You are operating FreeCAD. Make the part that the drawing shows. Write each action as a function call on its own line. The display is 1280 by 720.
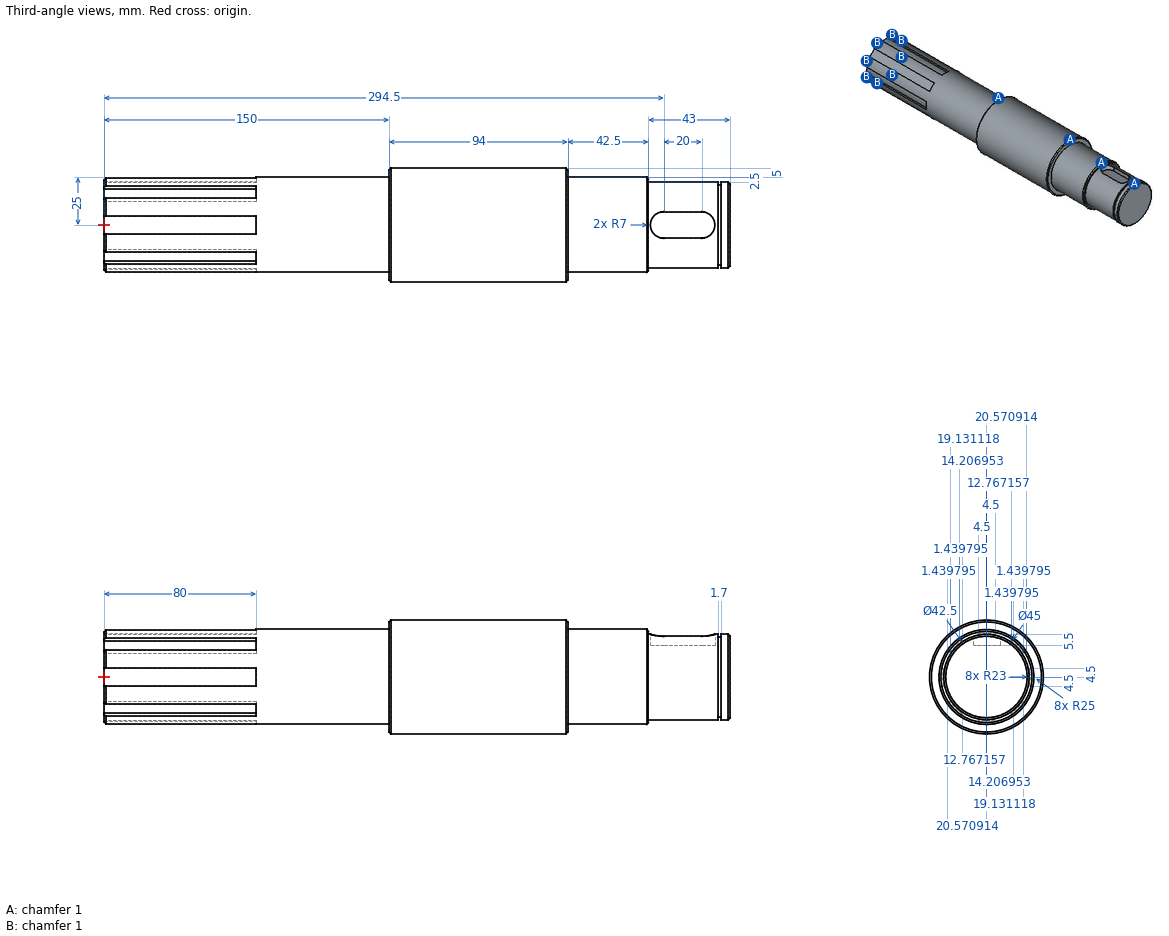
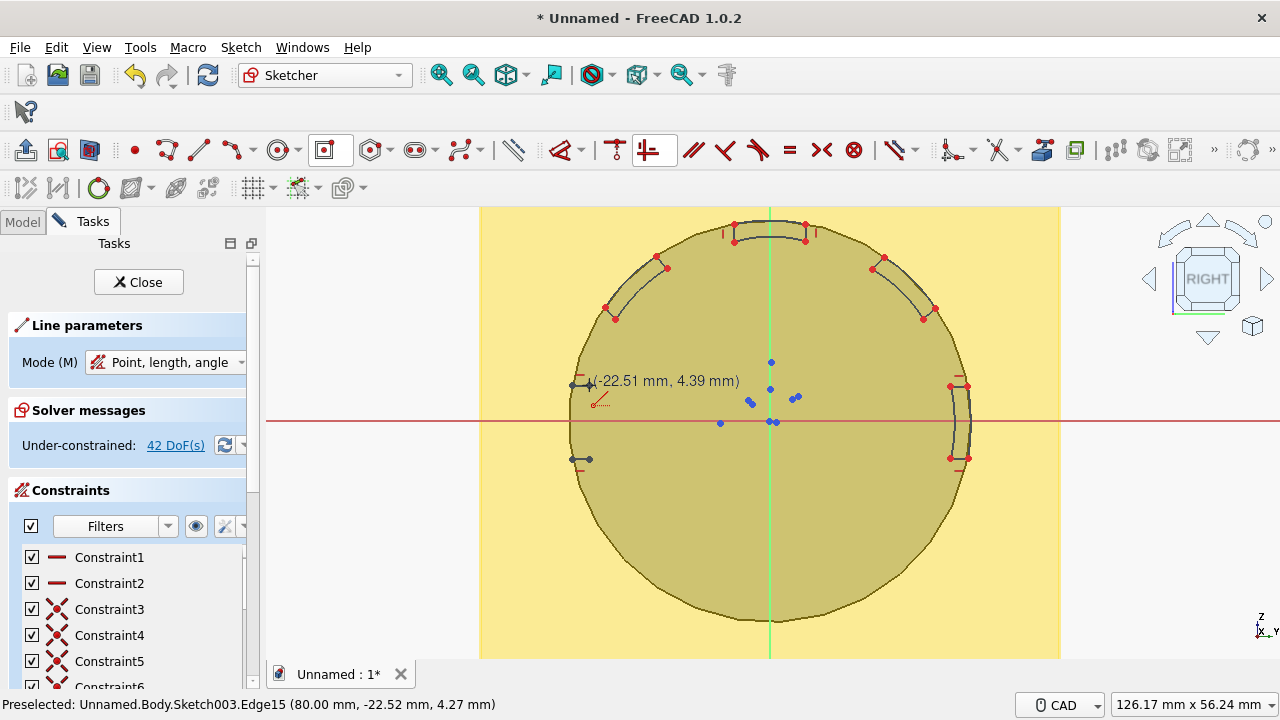
click(232, 150)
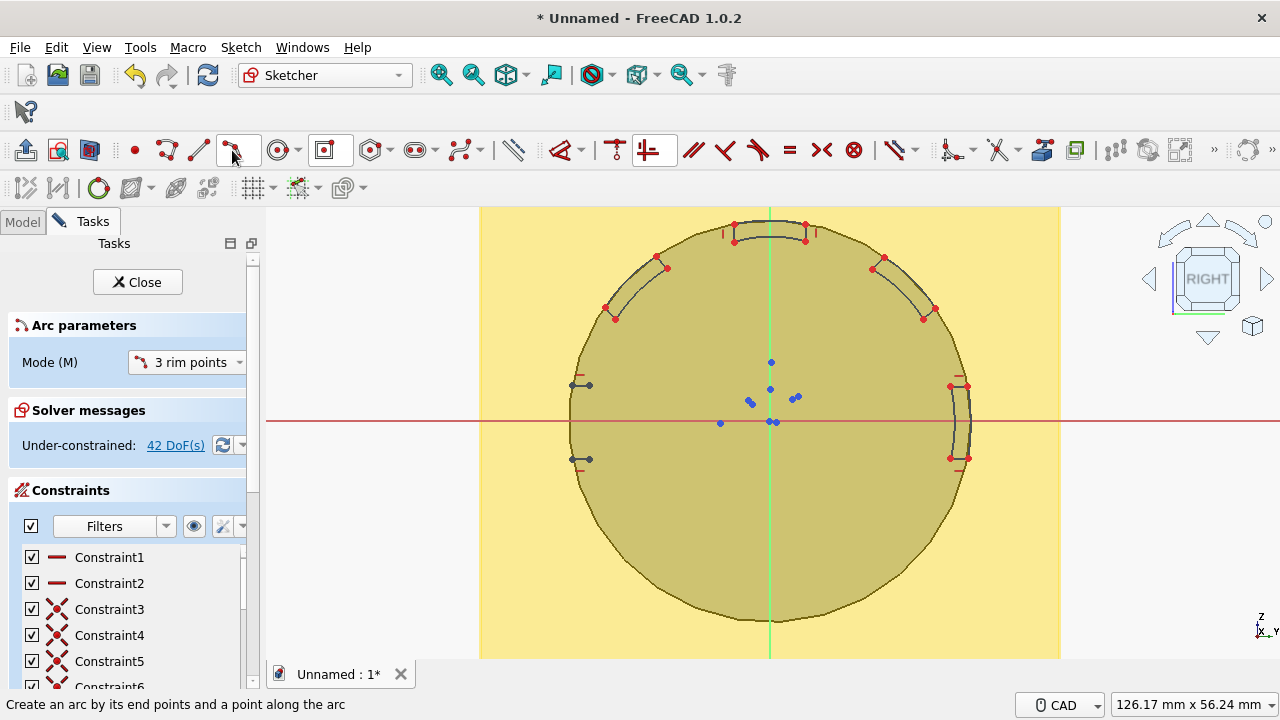
scroll(572, 457, up, 4)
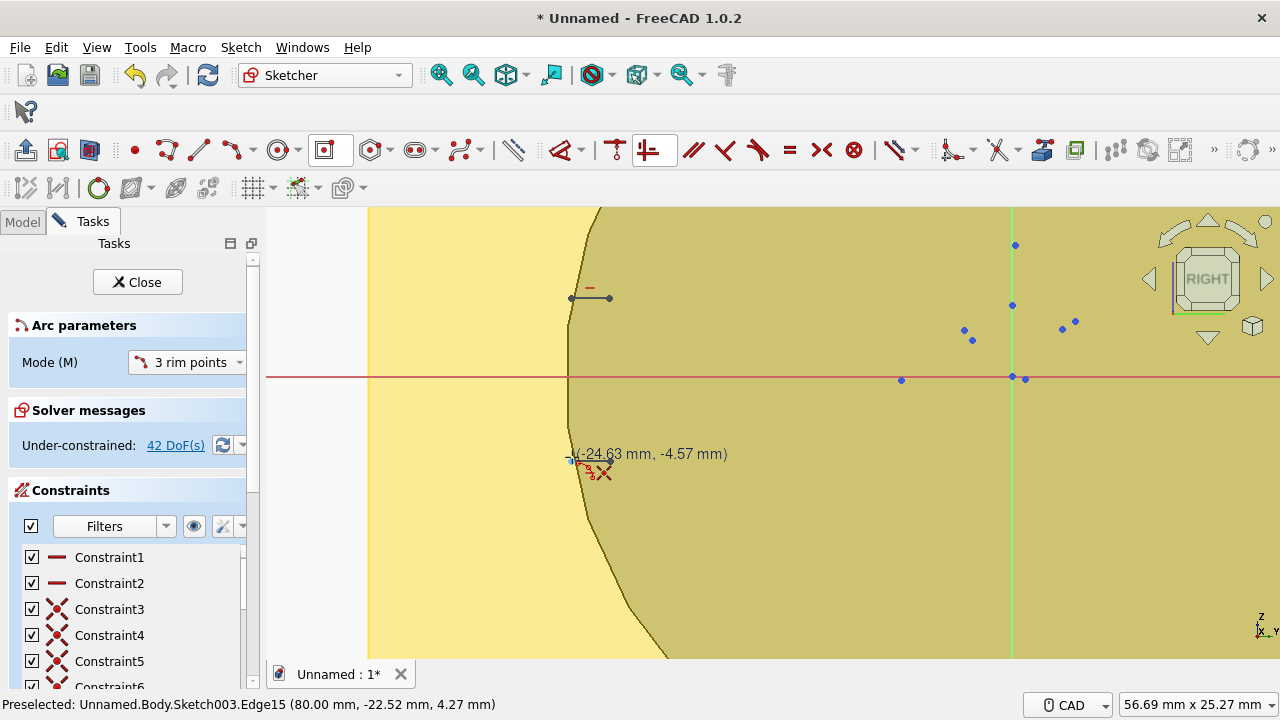
click(572, 461)
click(572, 298)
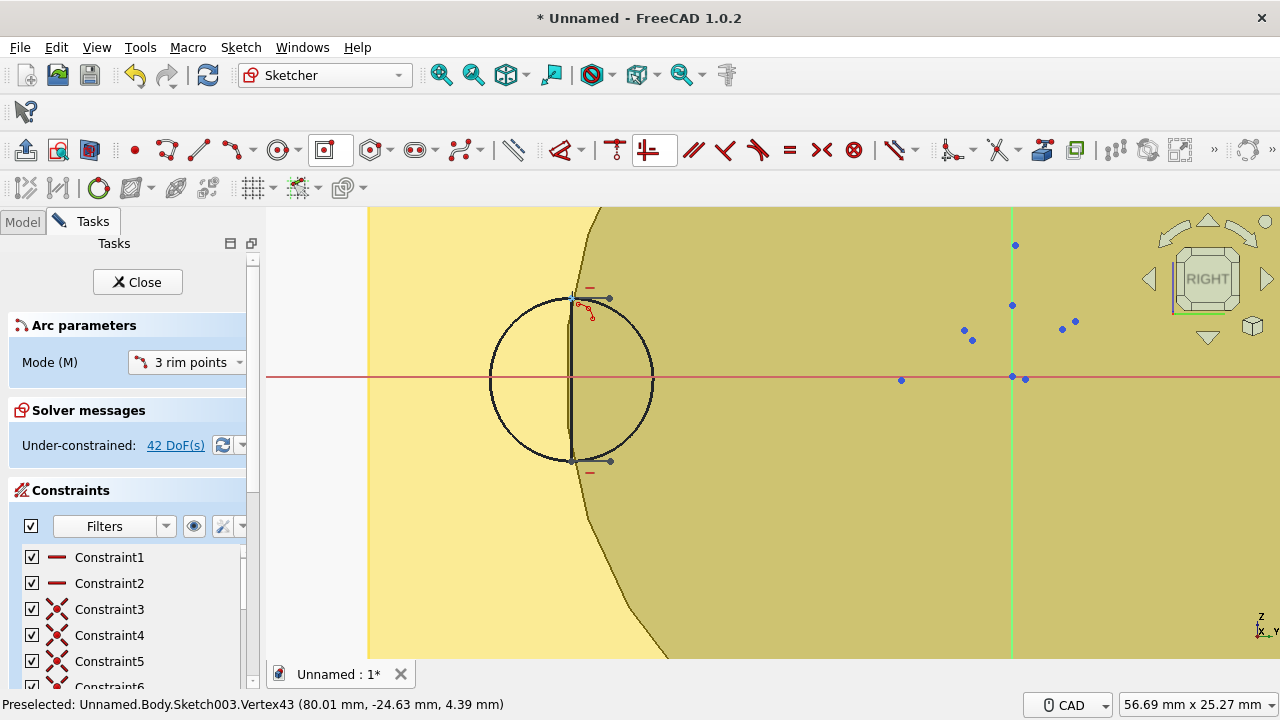
scroll(565, 361, up, 5)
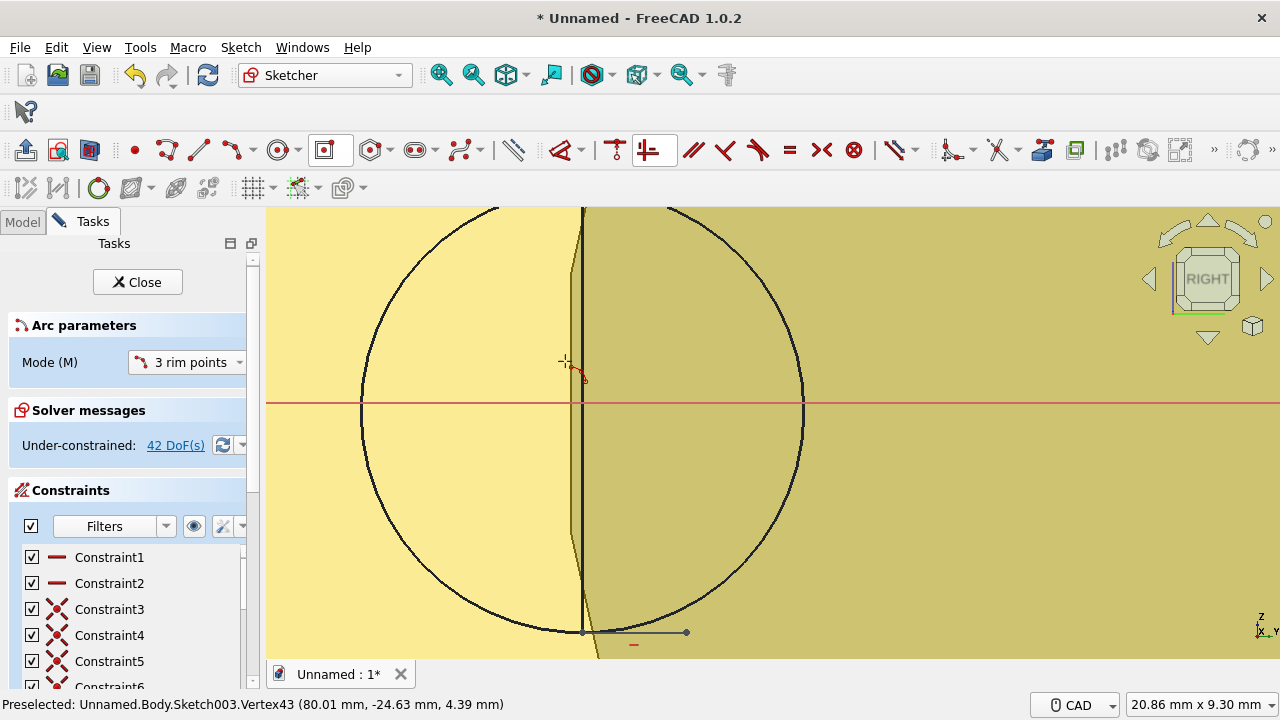
click(565, 359)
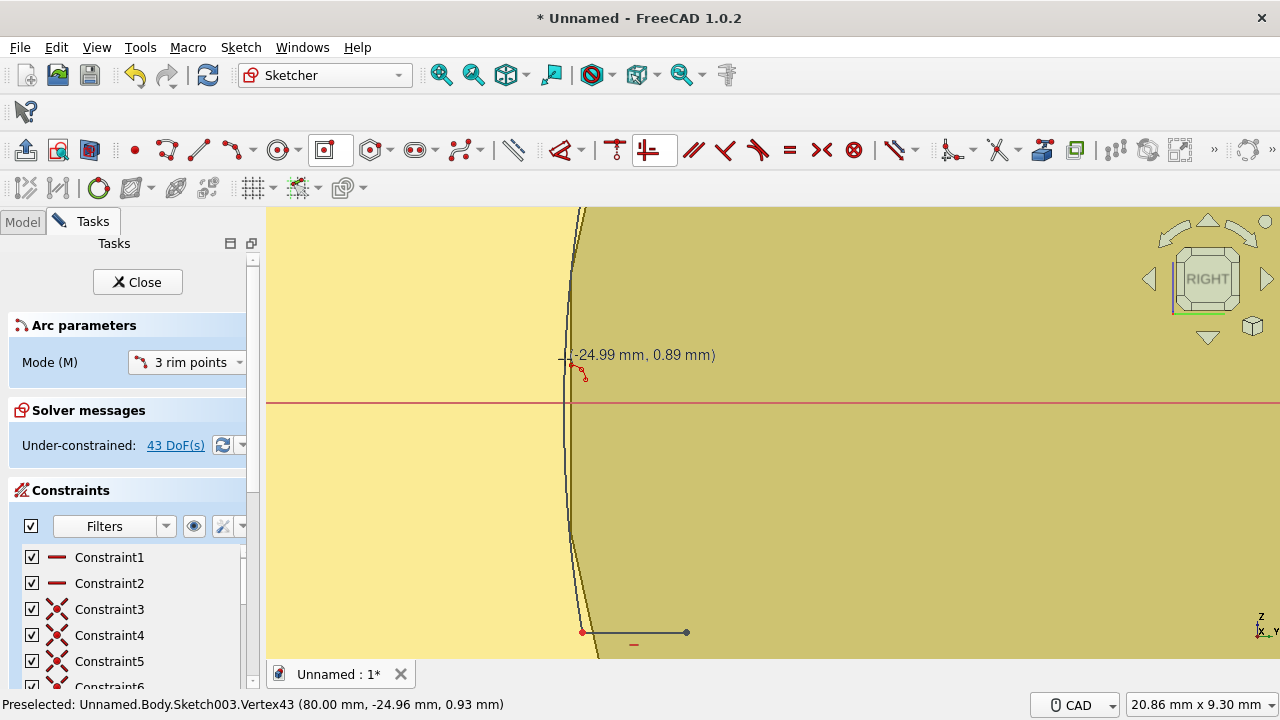
scroll(571, 437, down, 11)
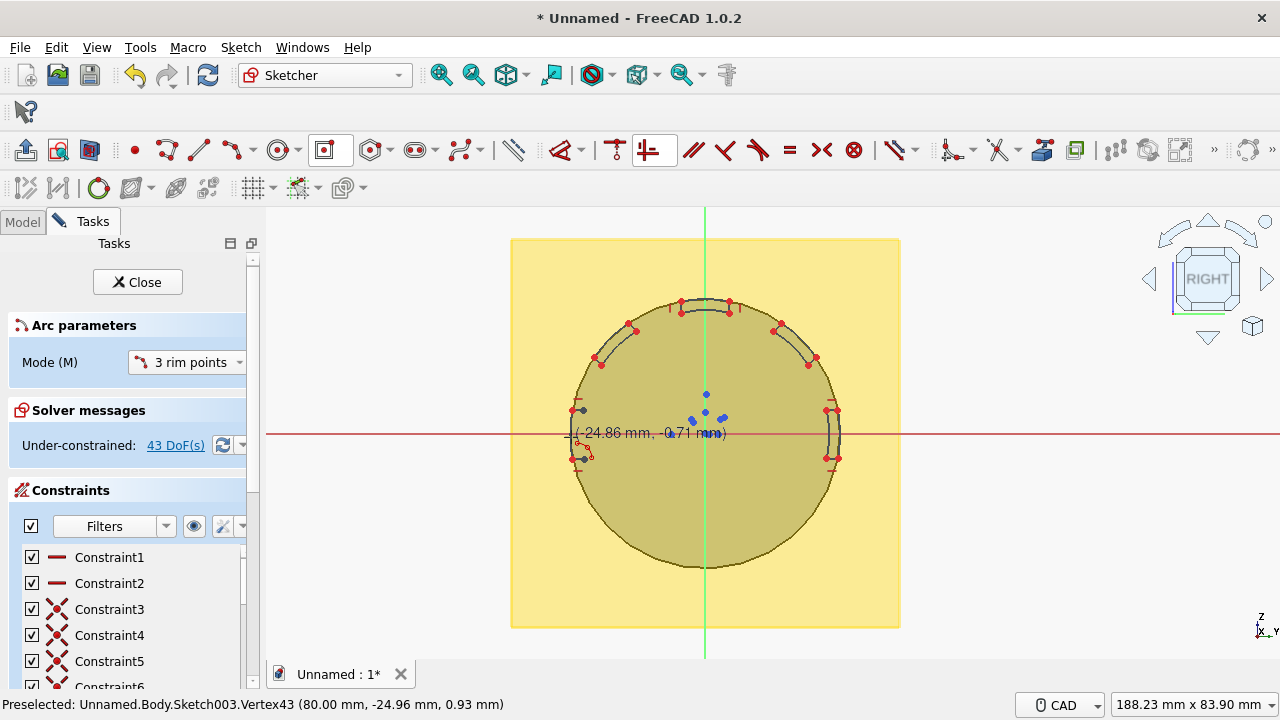
scroll(584, 409, up, 6)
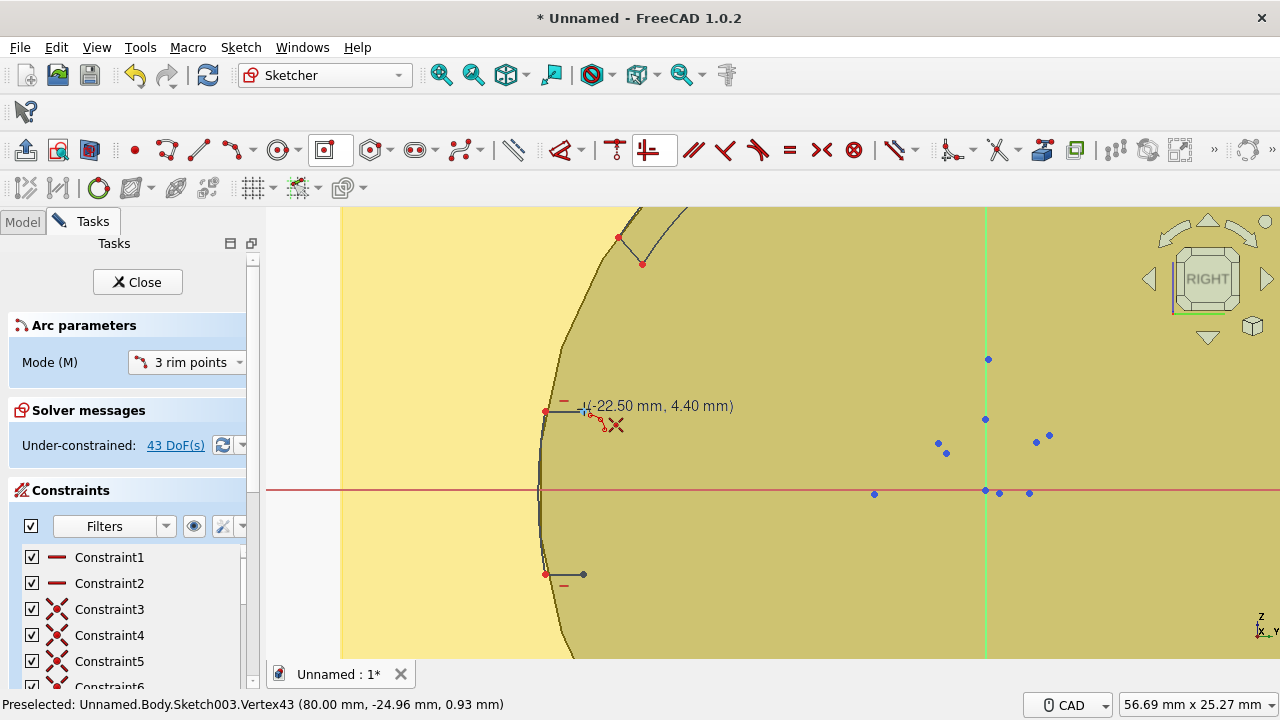
click(583, 412)
click(584, 575)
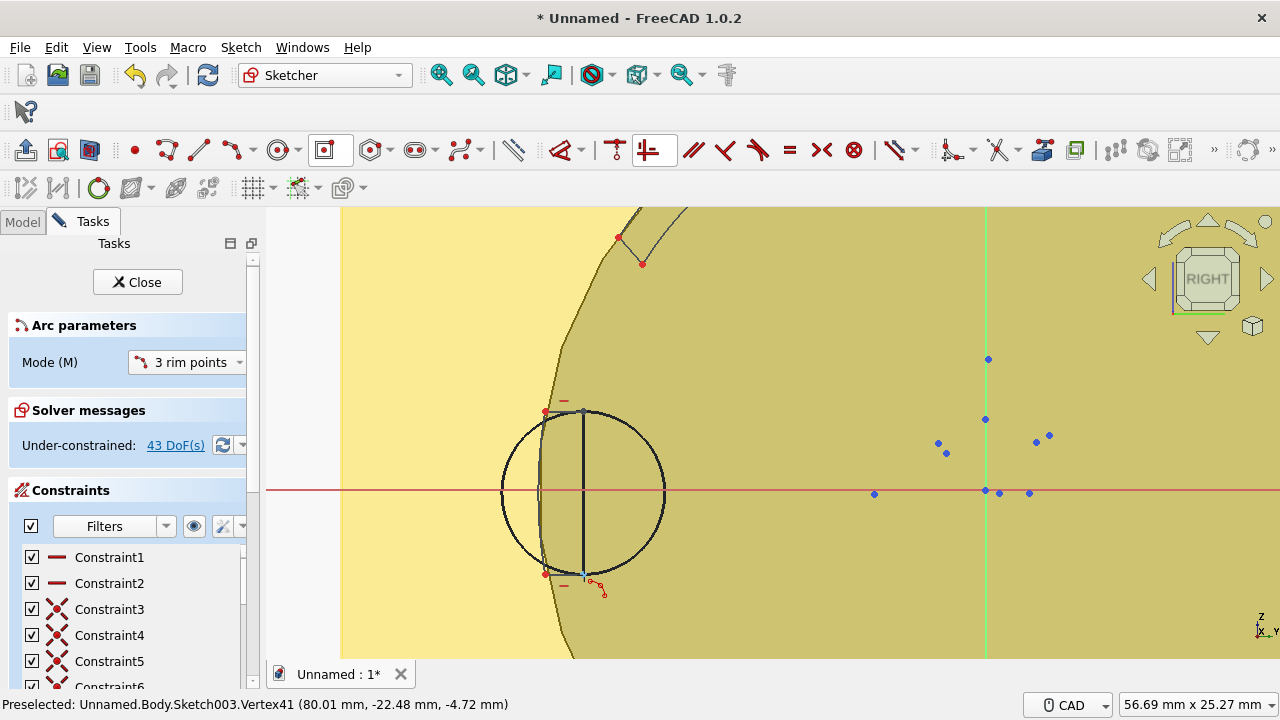
scroll(575, 474, up, 4)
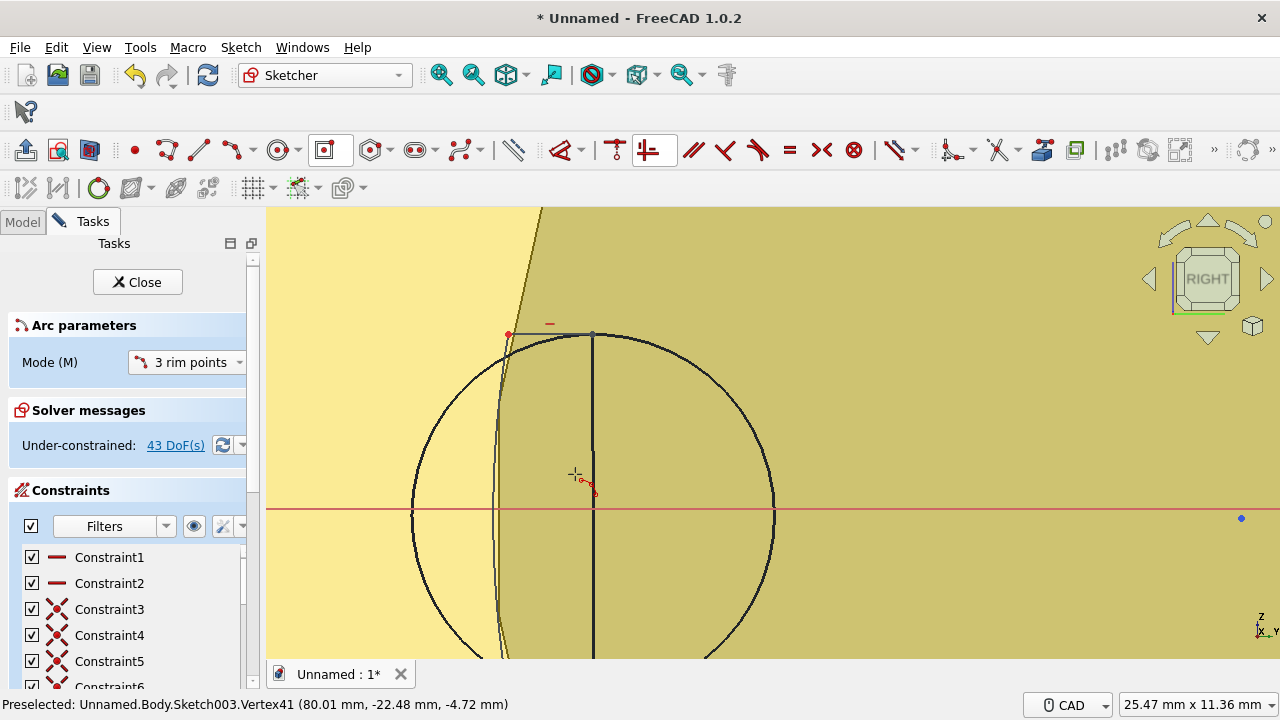
click(574, 473)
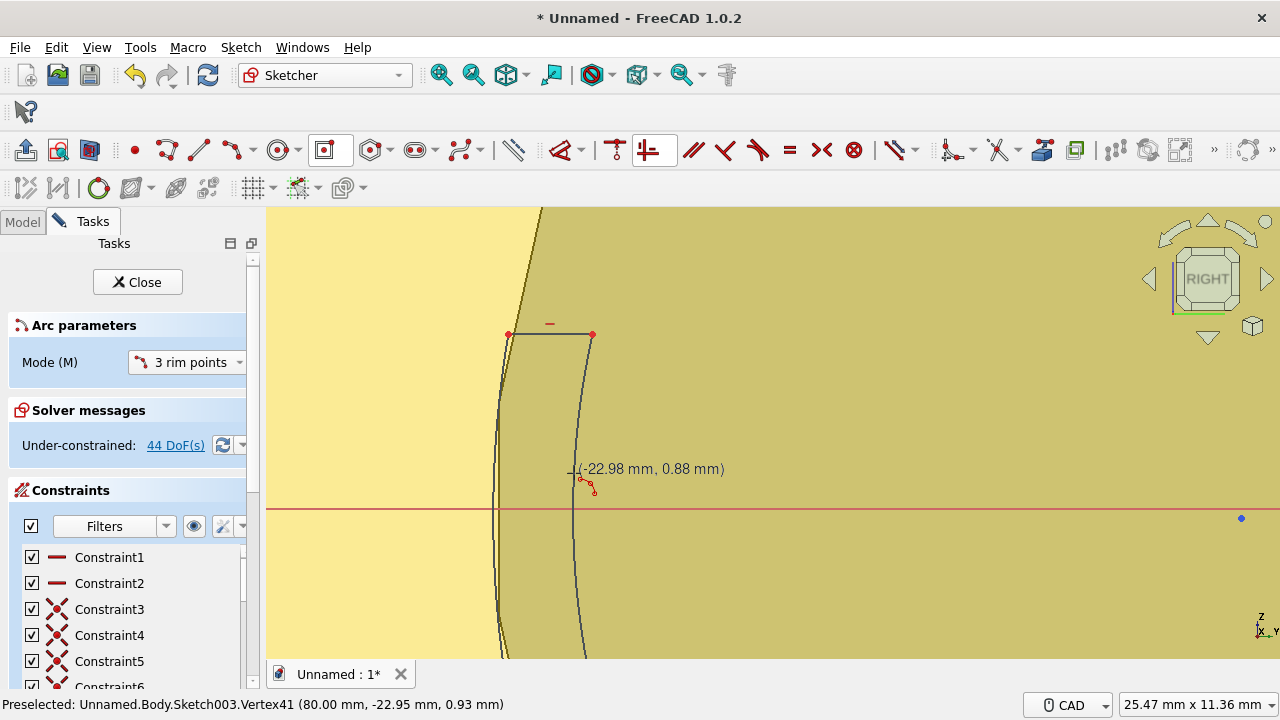
click(200, 150)